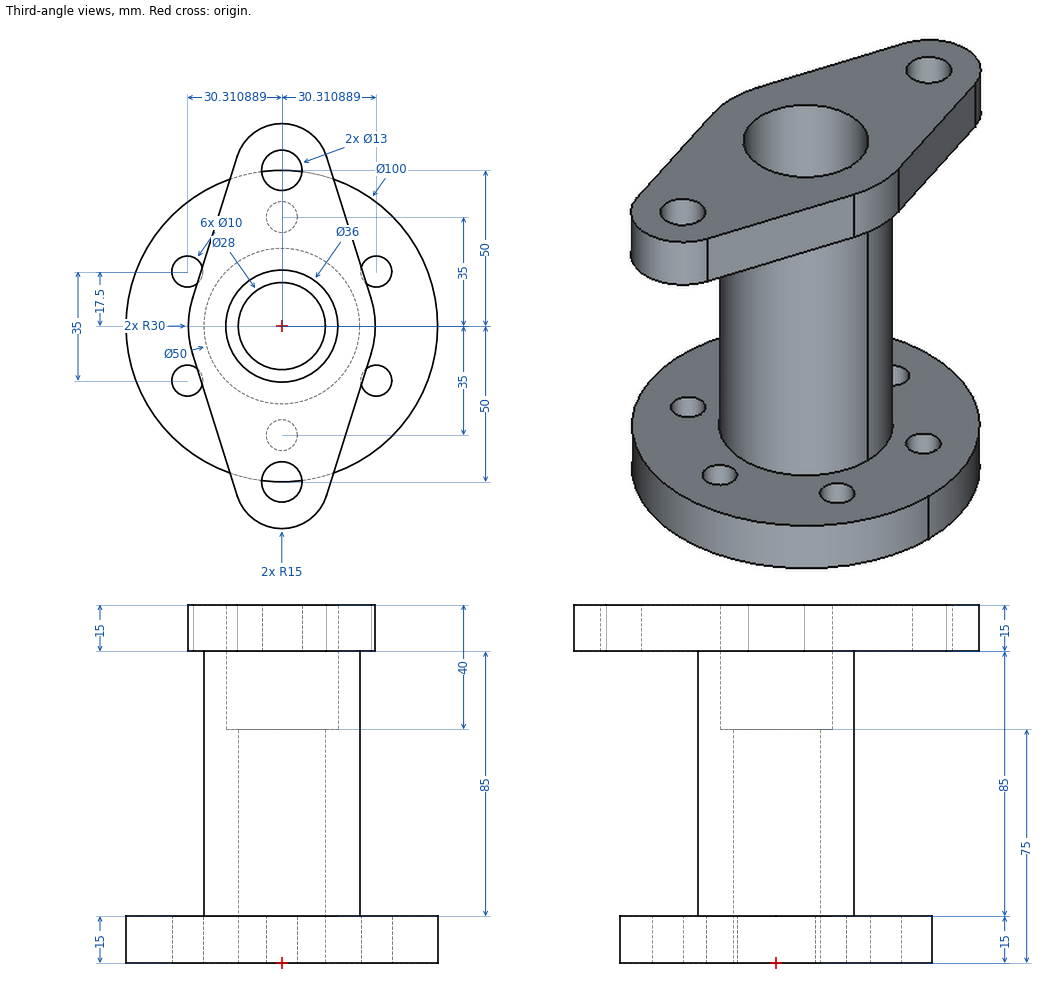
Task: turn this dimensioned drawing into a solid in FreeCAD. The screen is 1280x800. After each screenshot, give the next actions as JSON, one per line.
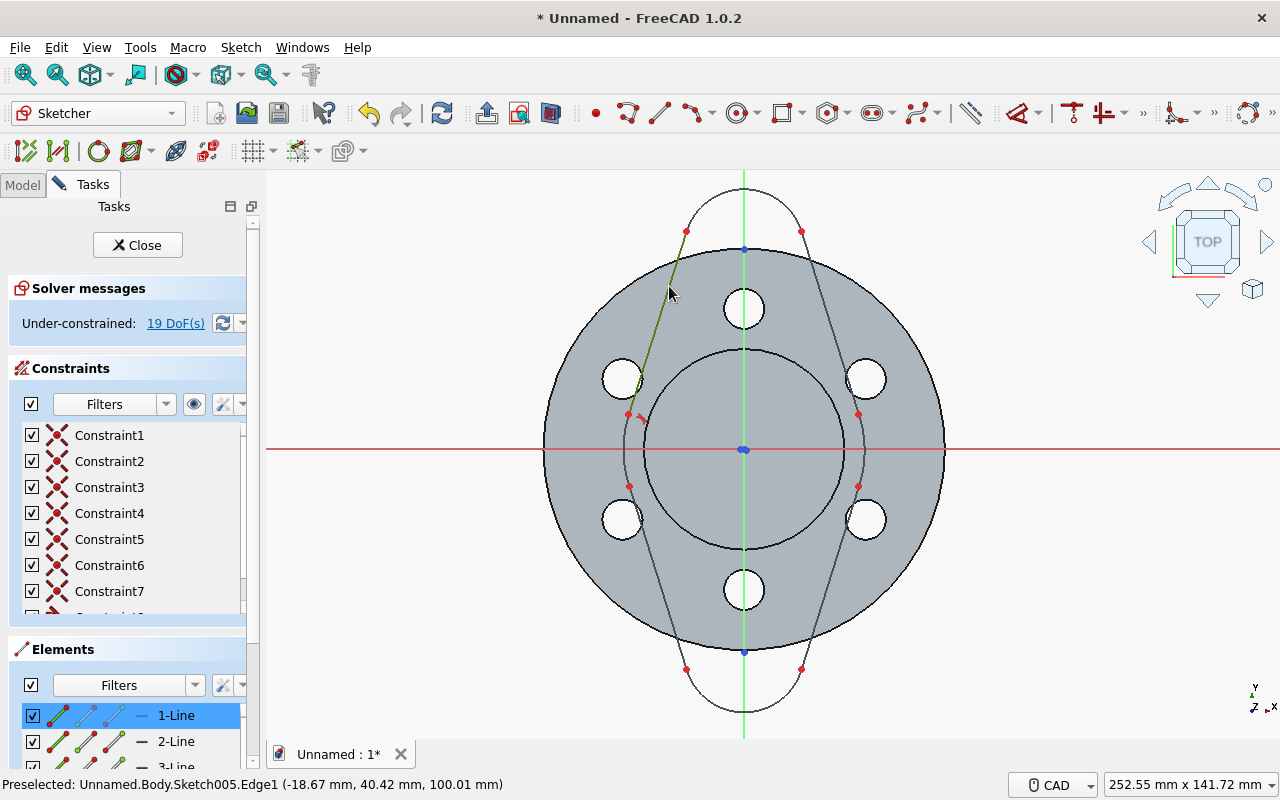
{"action": "left_click", "coordinate": [786, 206]}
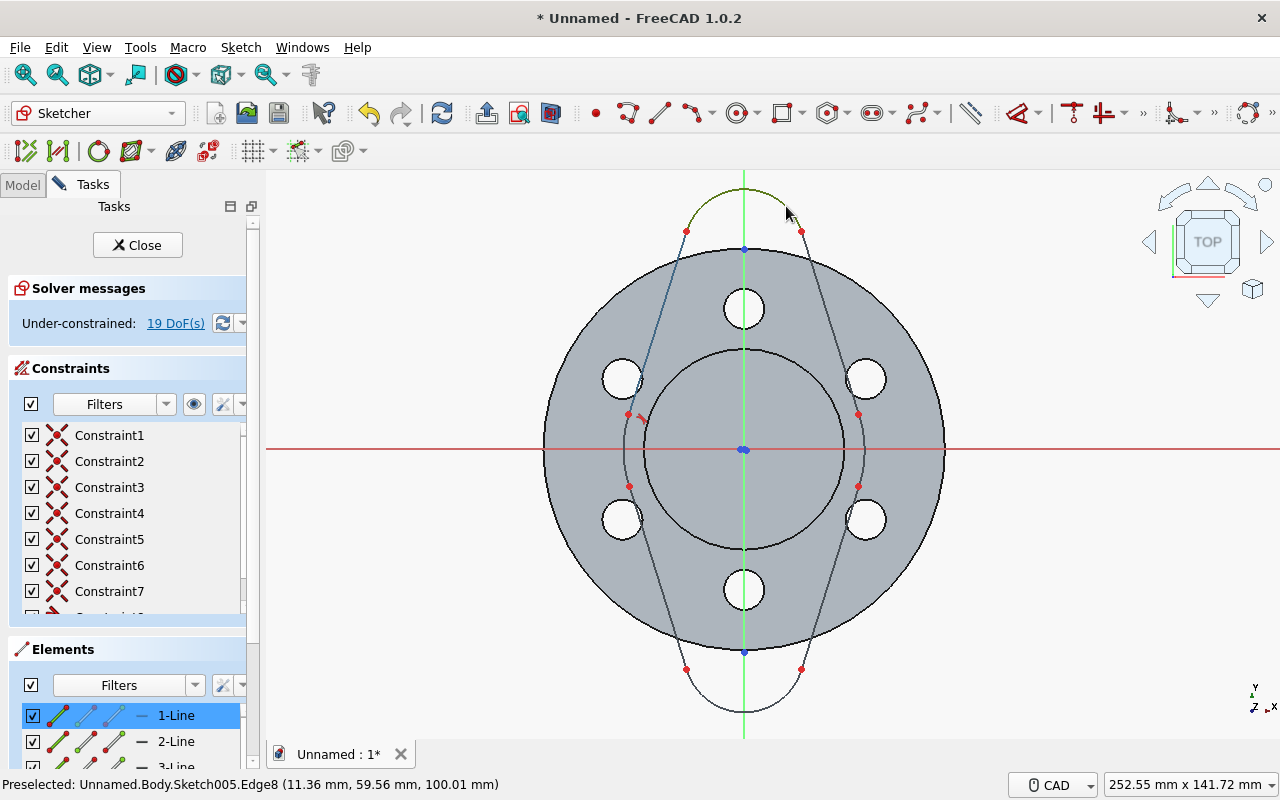
{"action": "key", "text": "t"}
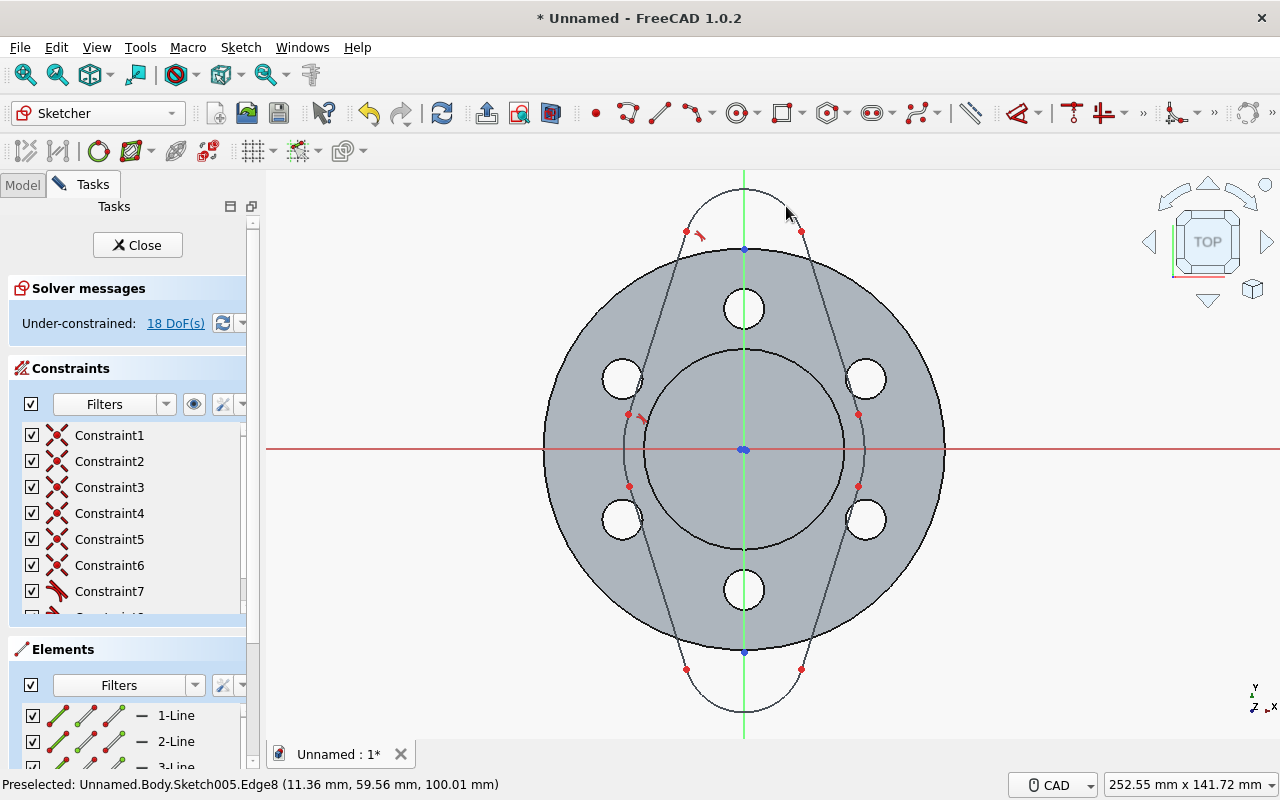
{"action": "left_click", "coordinate": [647, 542]}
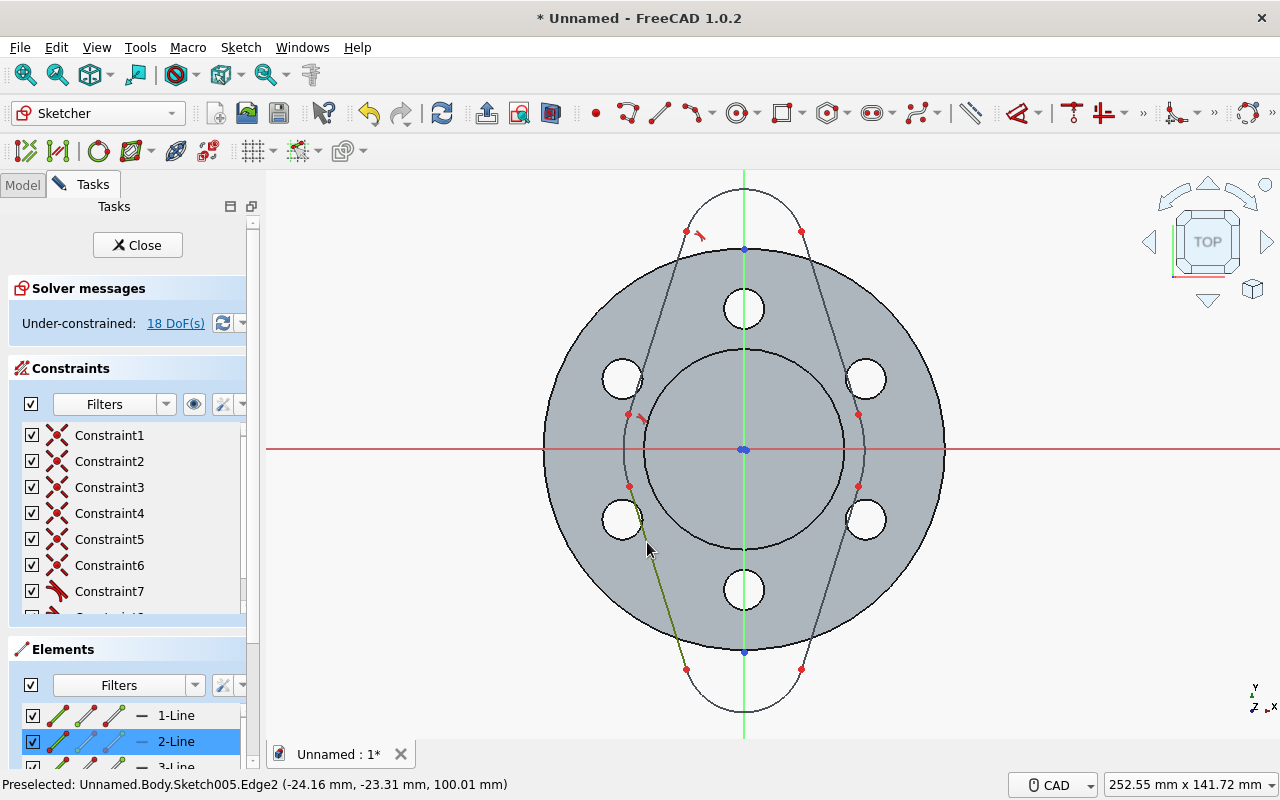
{"action": "left_click", "coordinate": [624, 436]}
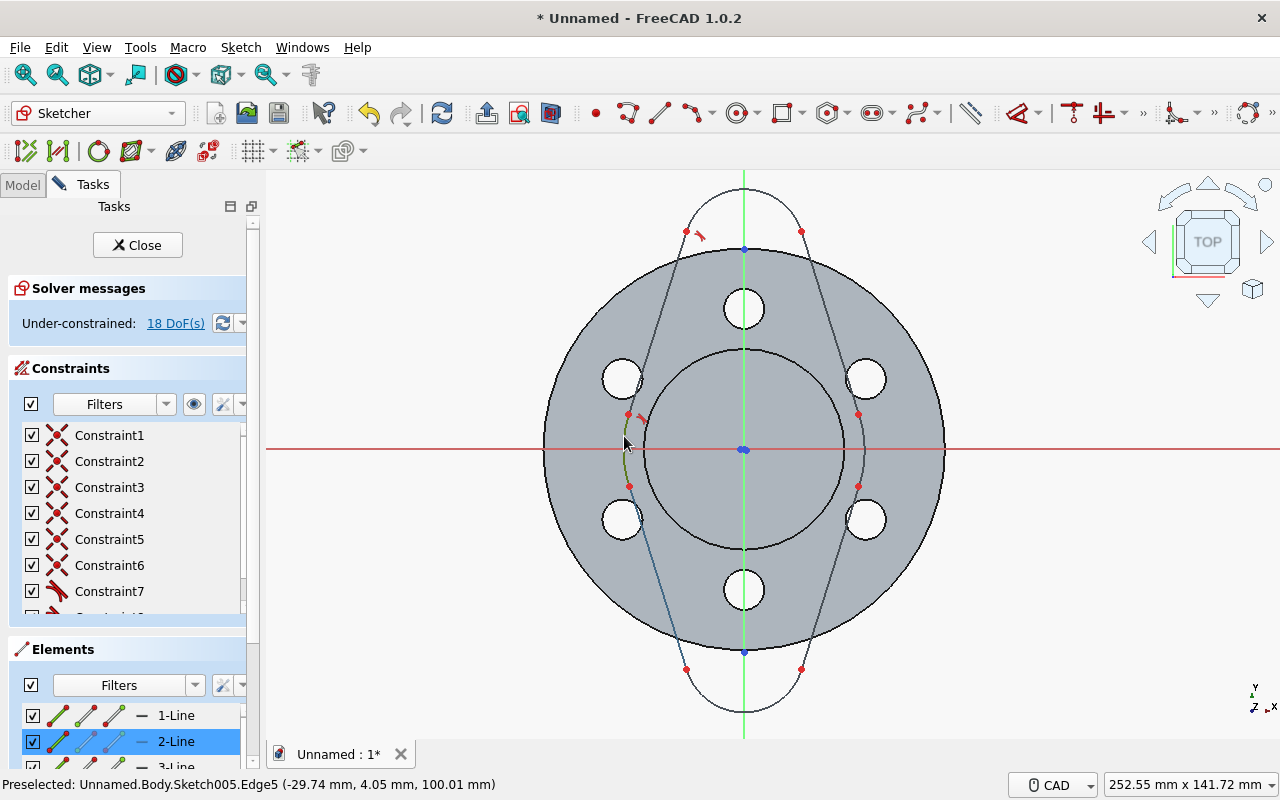
{"action": "key", "text": "t"}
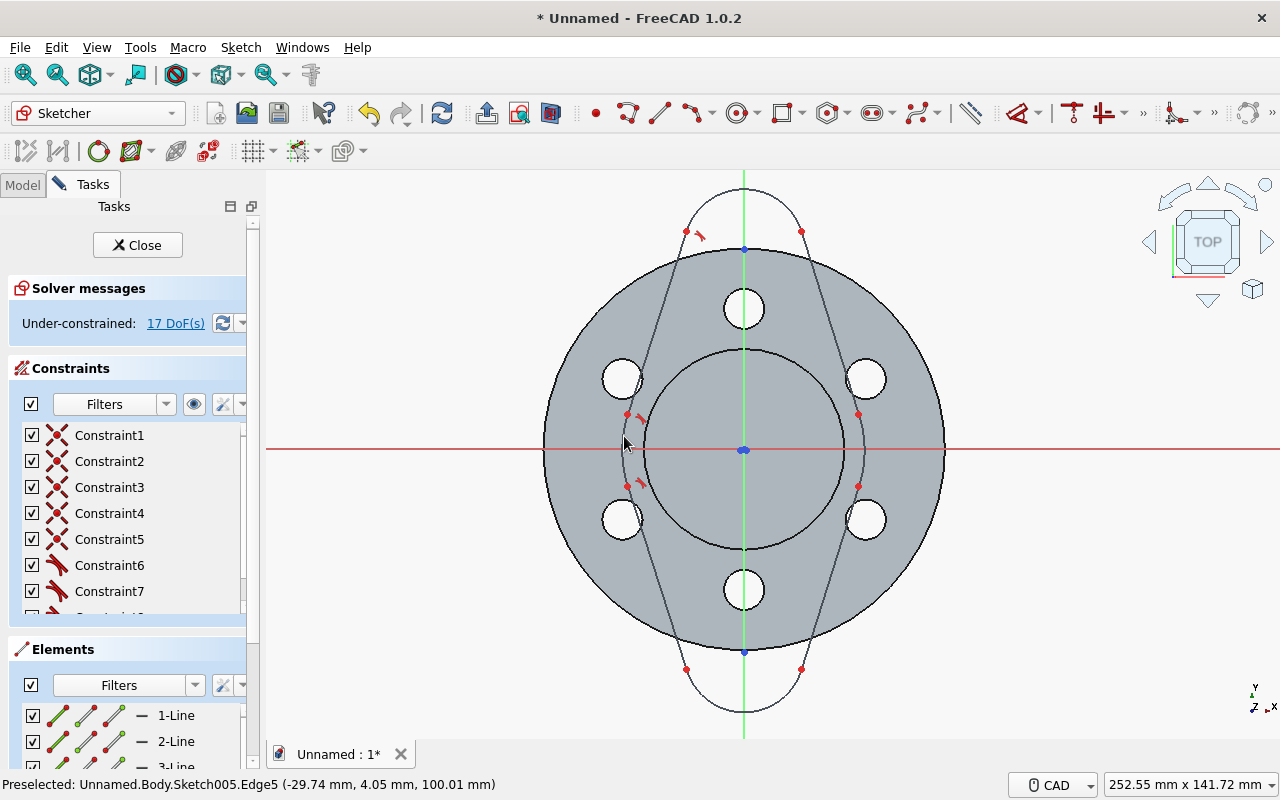
{"action": "left_click", "coordinate": [646, 542]}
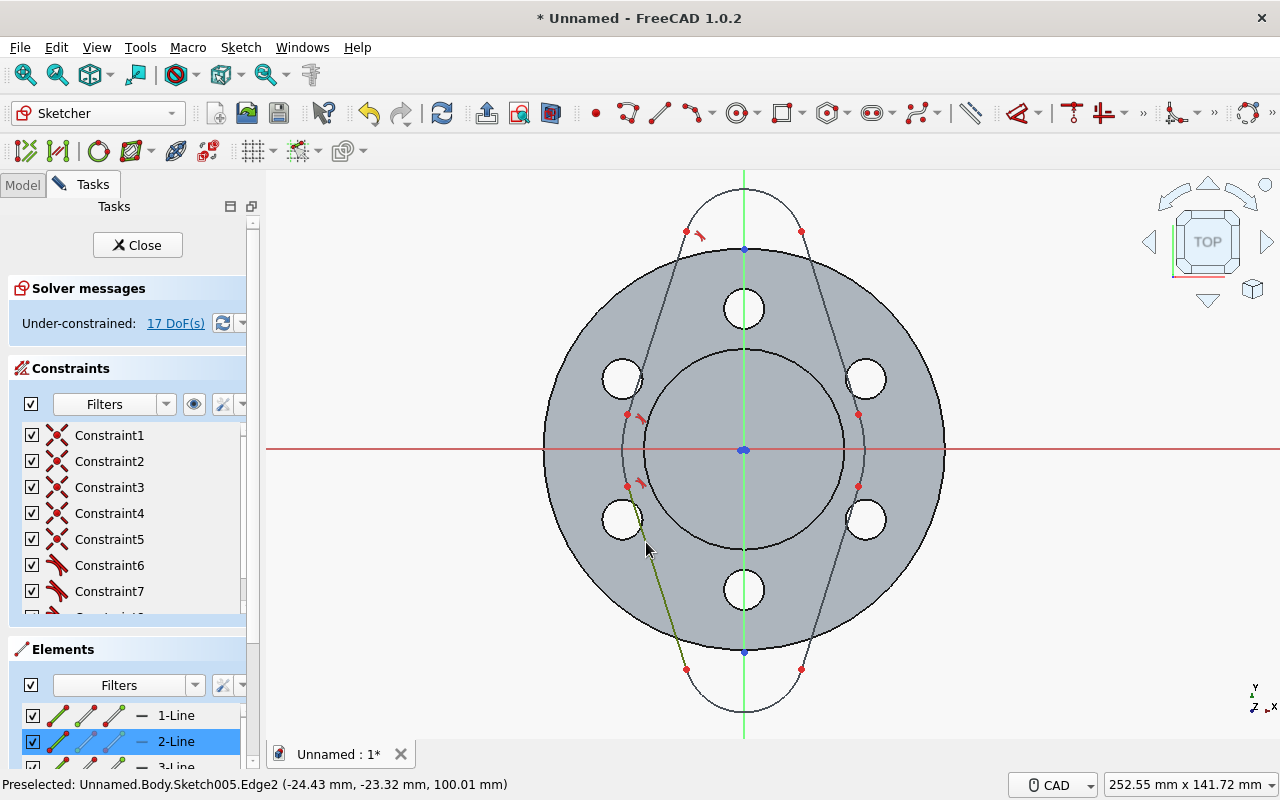
{"action": "left_click", "coordinate": [715, 705]}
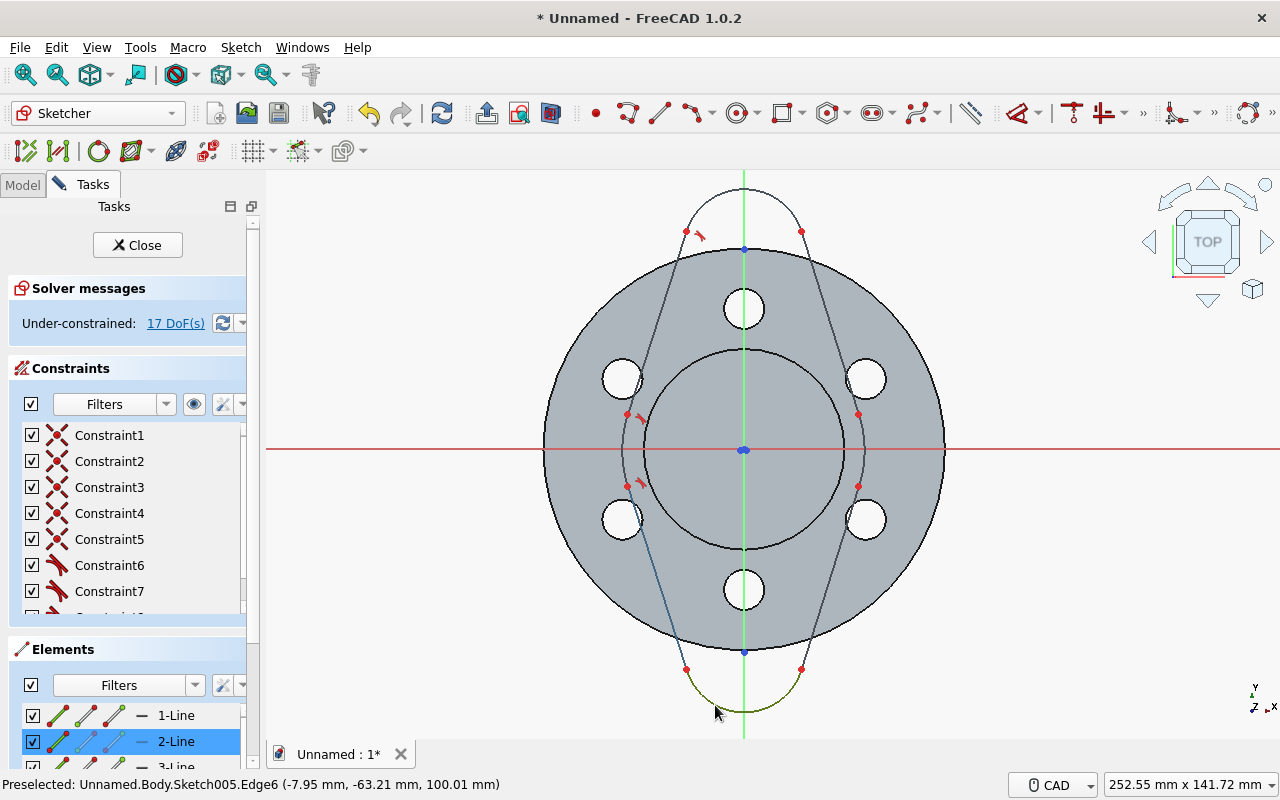
{"action": "key", "text": "t"}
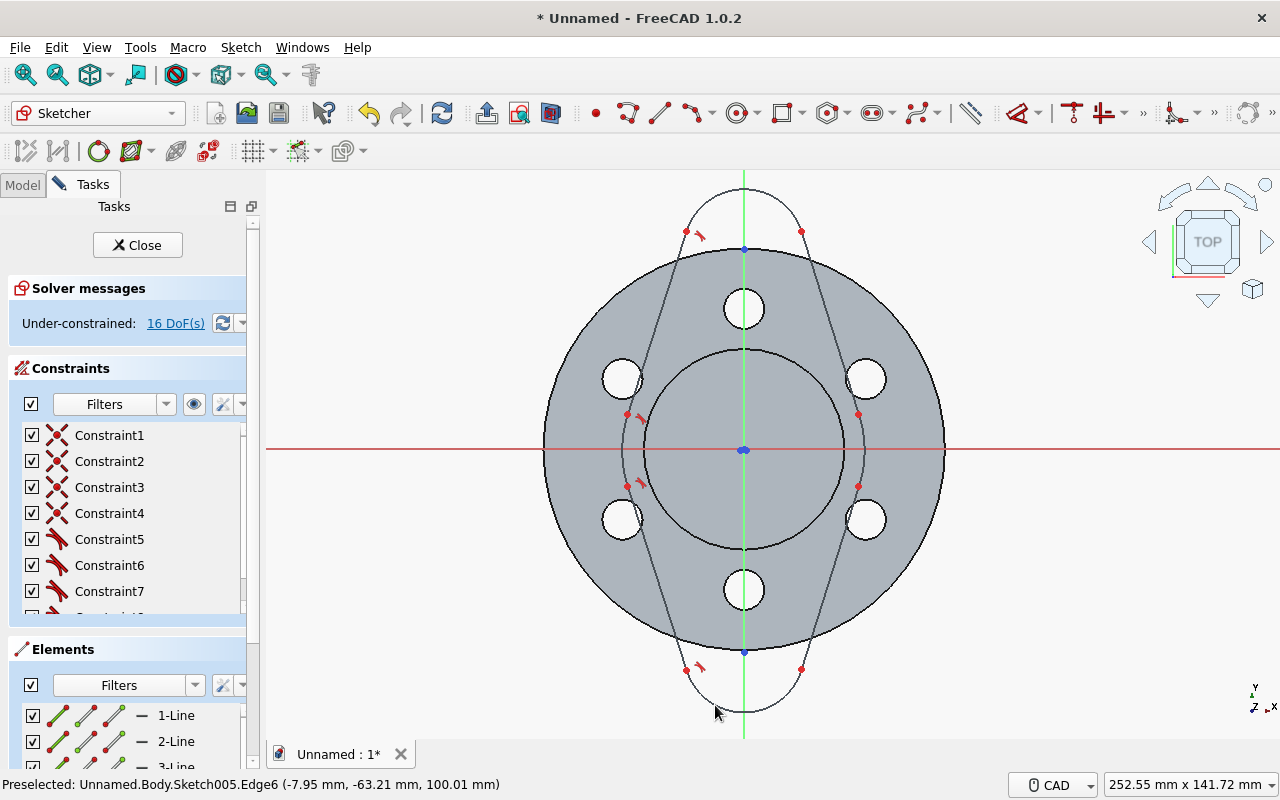
{"action": "left_click", "coordinate": [819, 615]}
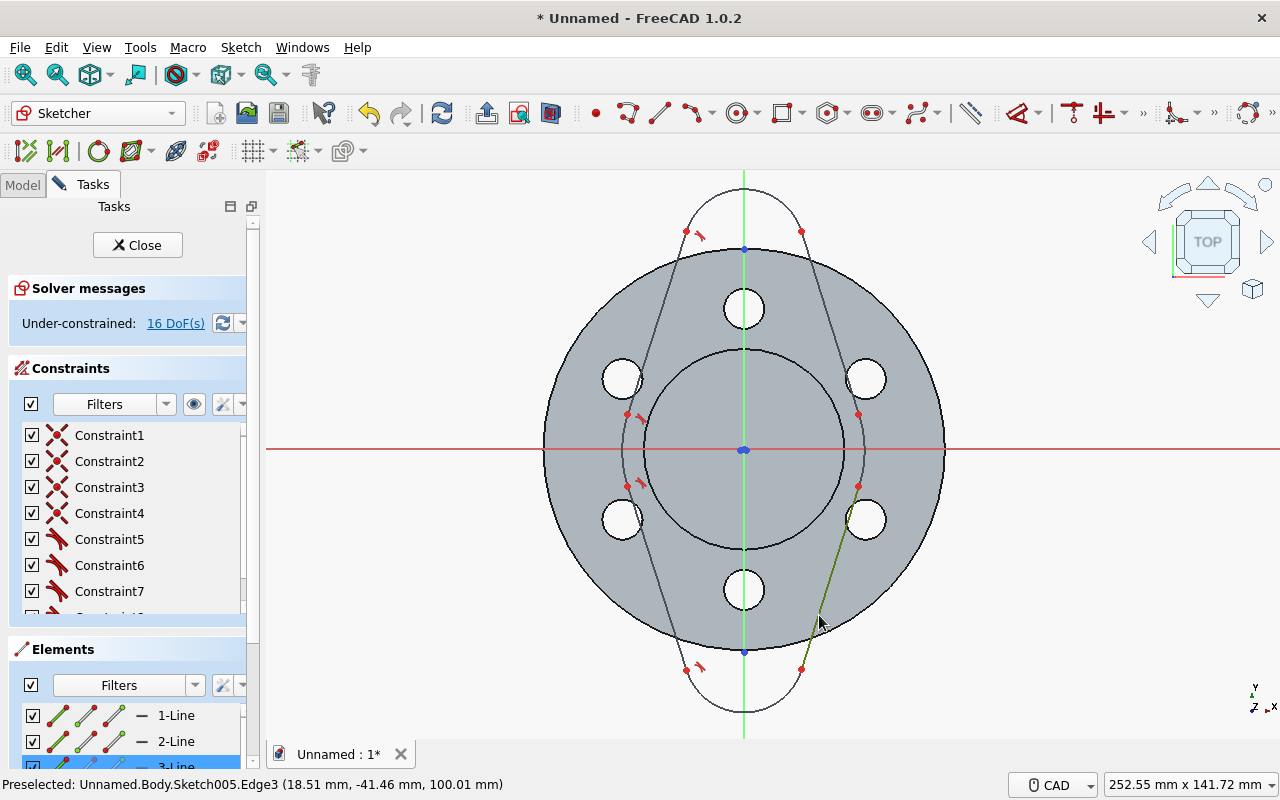
{"action": "left_click", "coordinate": [715, 705]}